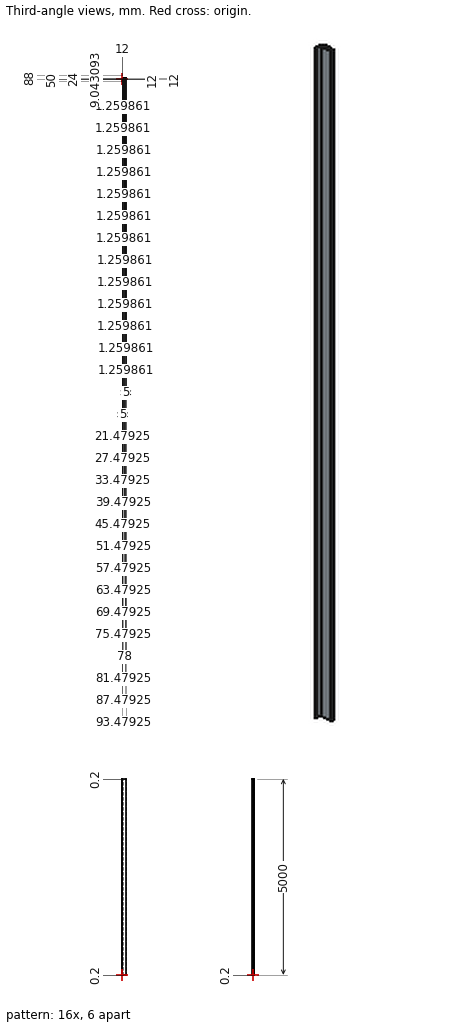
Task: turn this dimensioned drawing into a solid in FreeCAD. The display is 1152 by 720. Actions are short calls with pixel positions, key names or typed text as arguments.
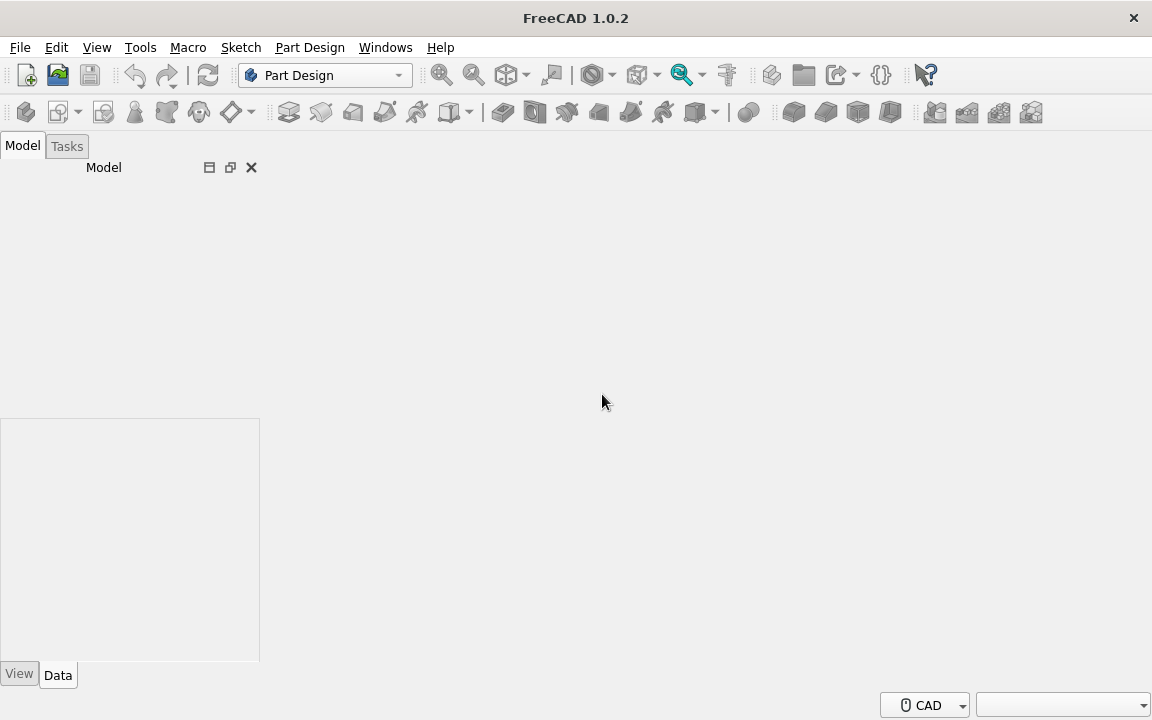
click(26, 76)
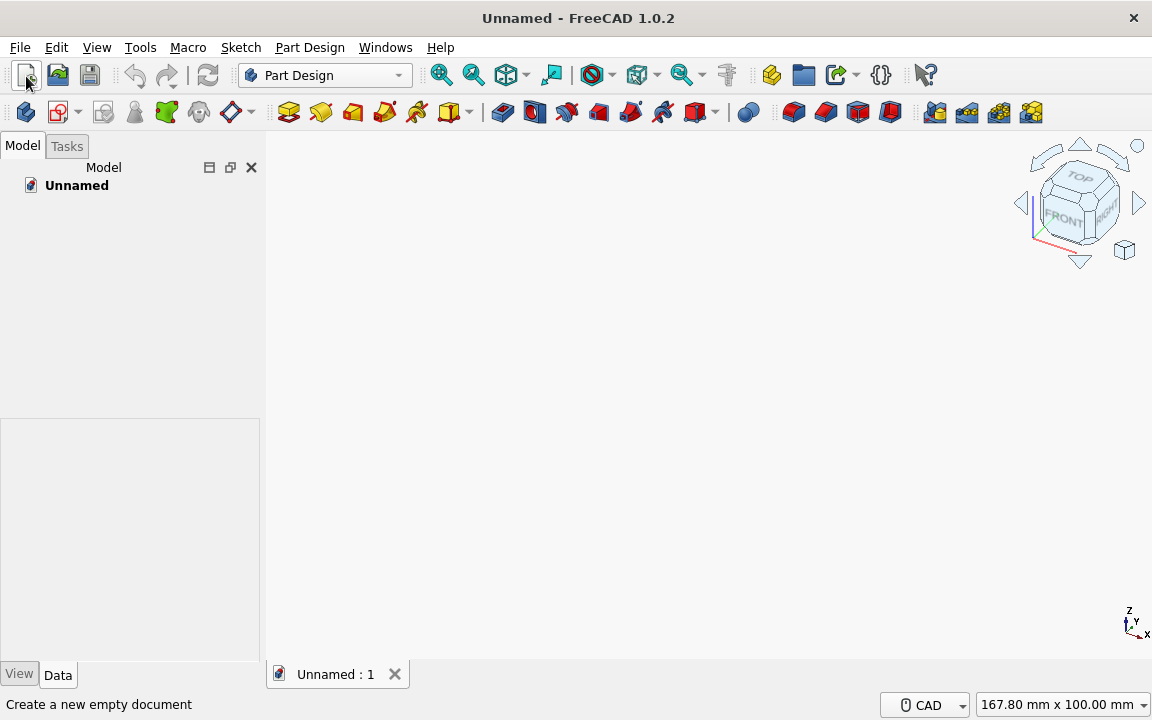
click(58, 112)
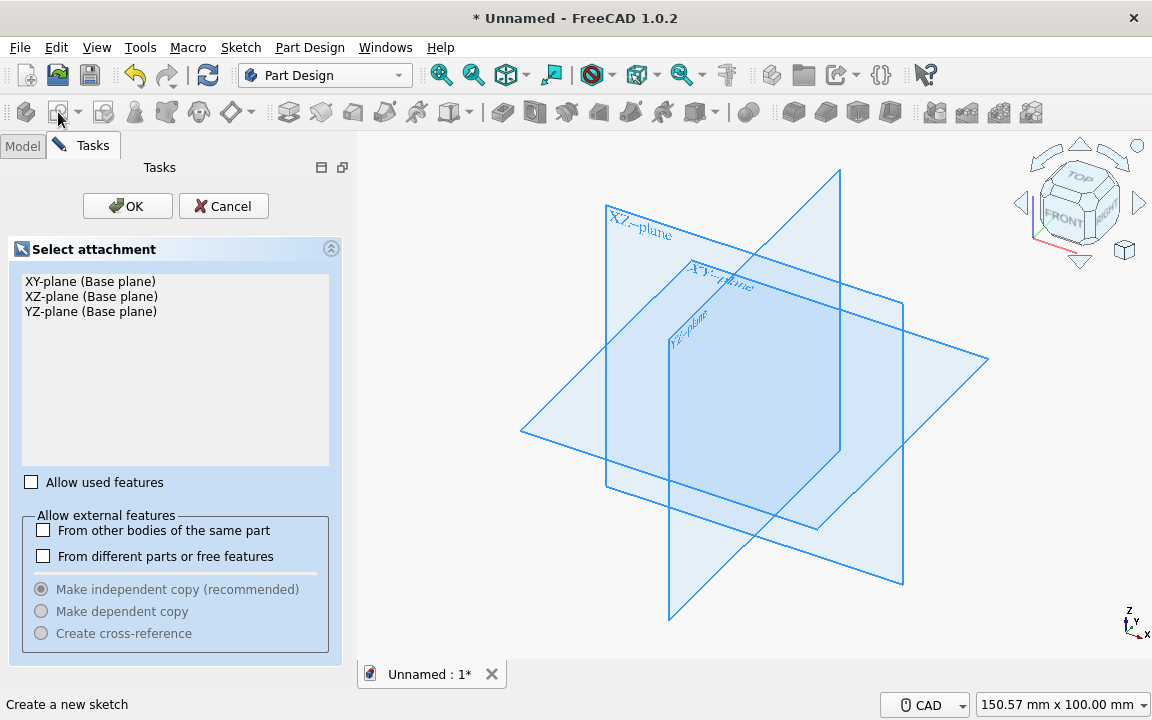
click(82, 282)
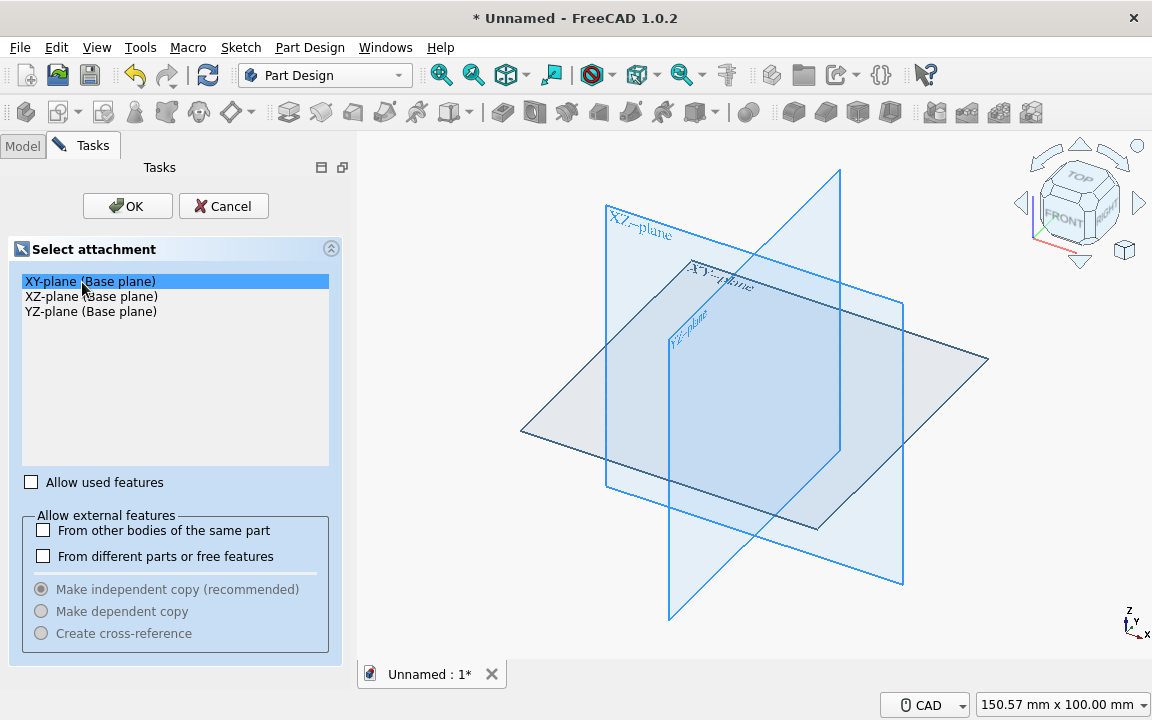
click(128, 206)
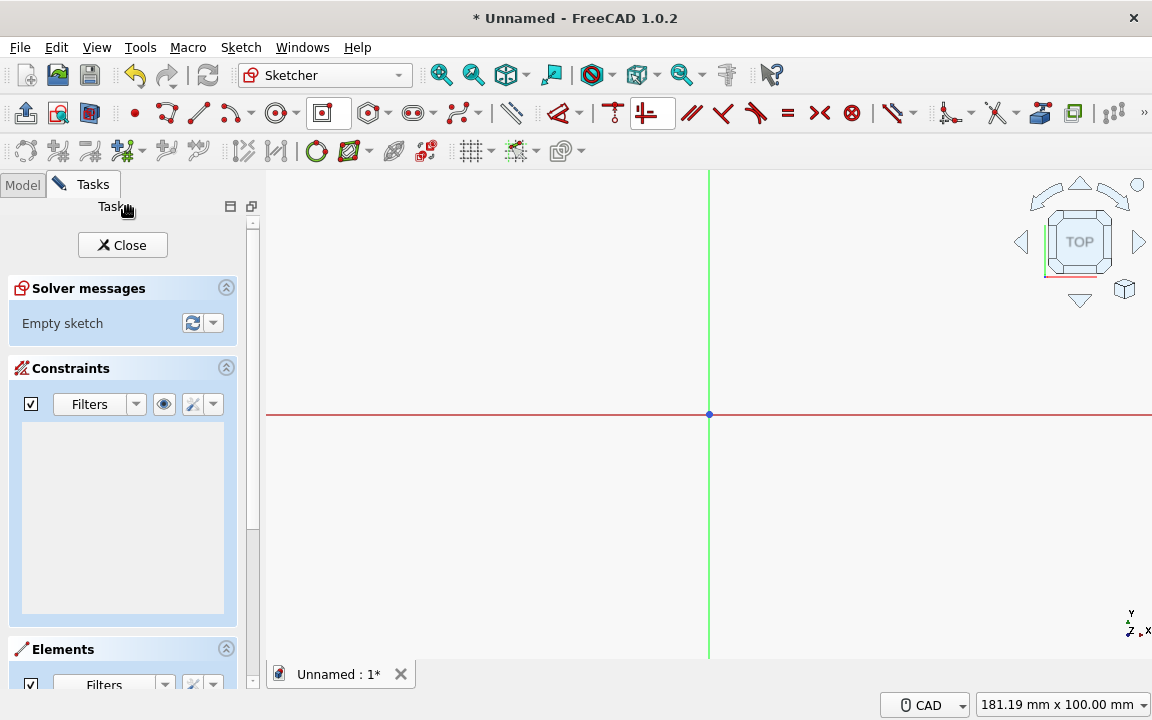
scroll(294, 631, down, 3)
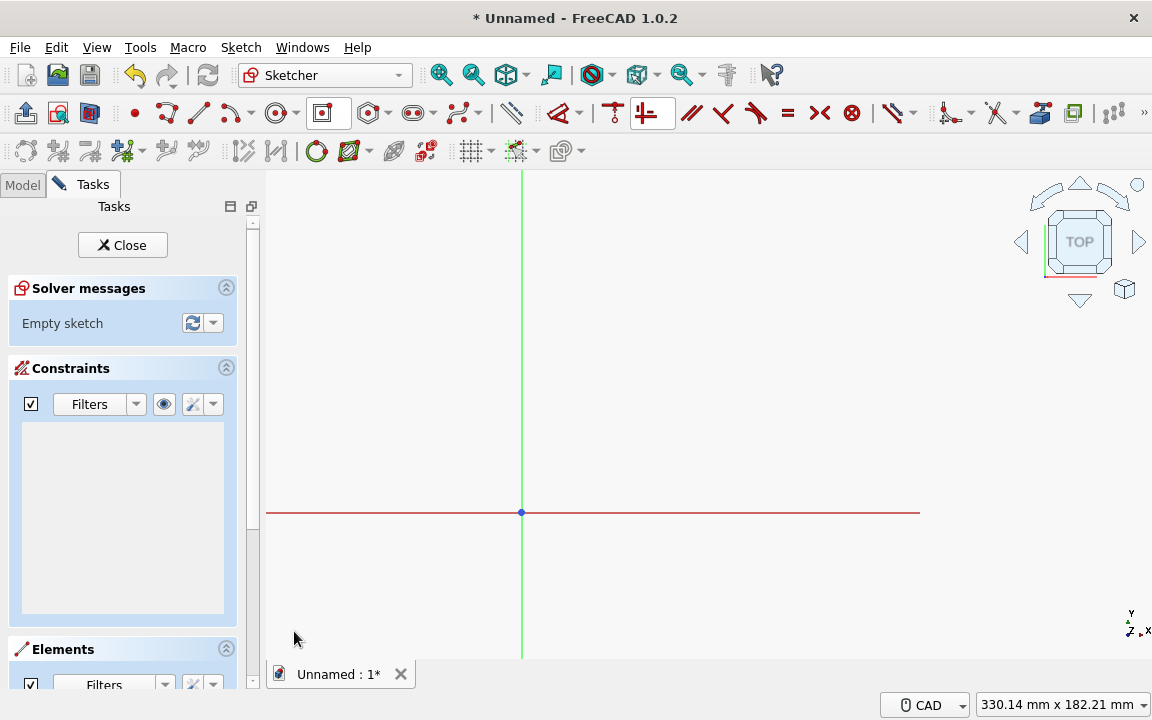
click(168, 114)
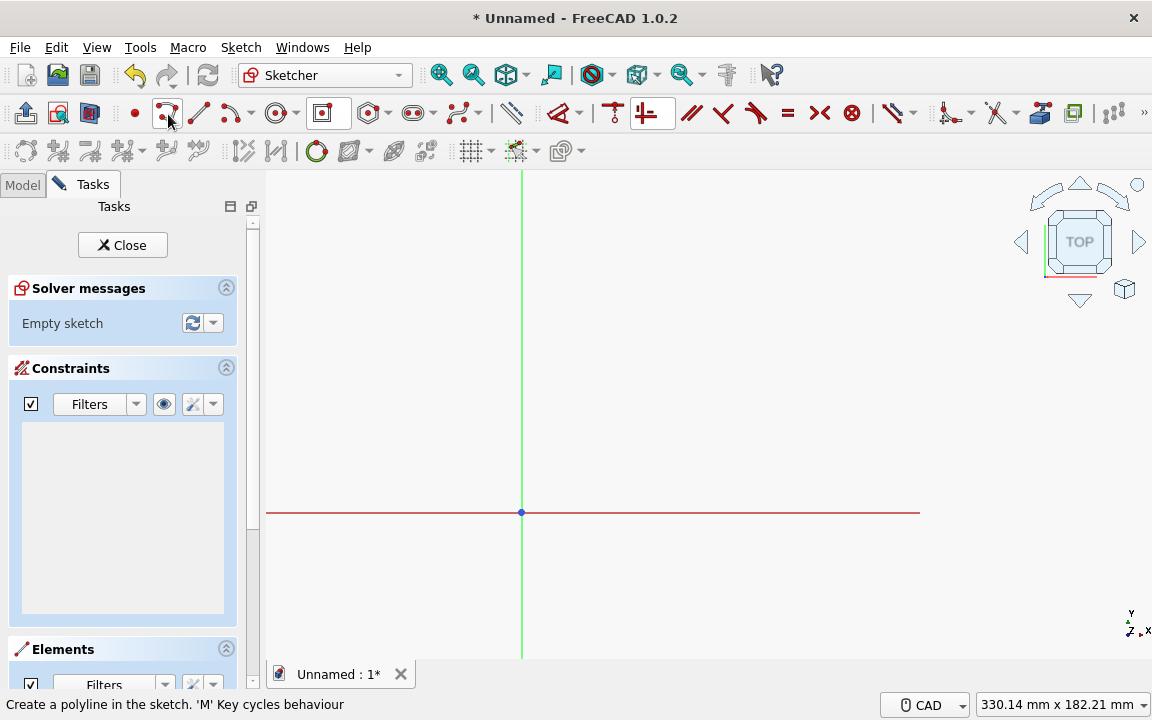
click(522, 513)
click(790, 504)
click(790, 480)
click(777, 480)
click(777, 448)
click(567, 448)
click(567, 480)
click(554, 480)
click(554, 244)
click(531, 244)
click(522, 513)
key(Escape)
key(Escape)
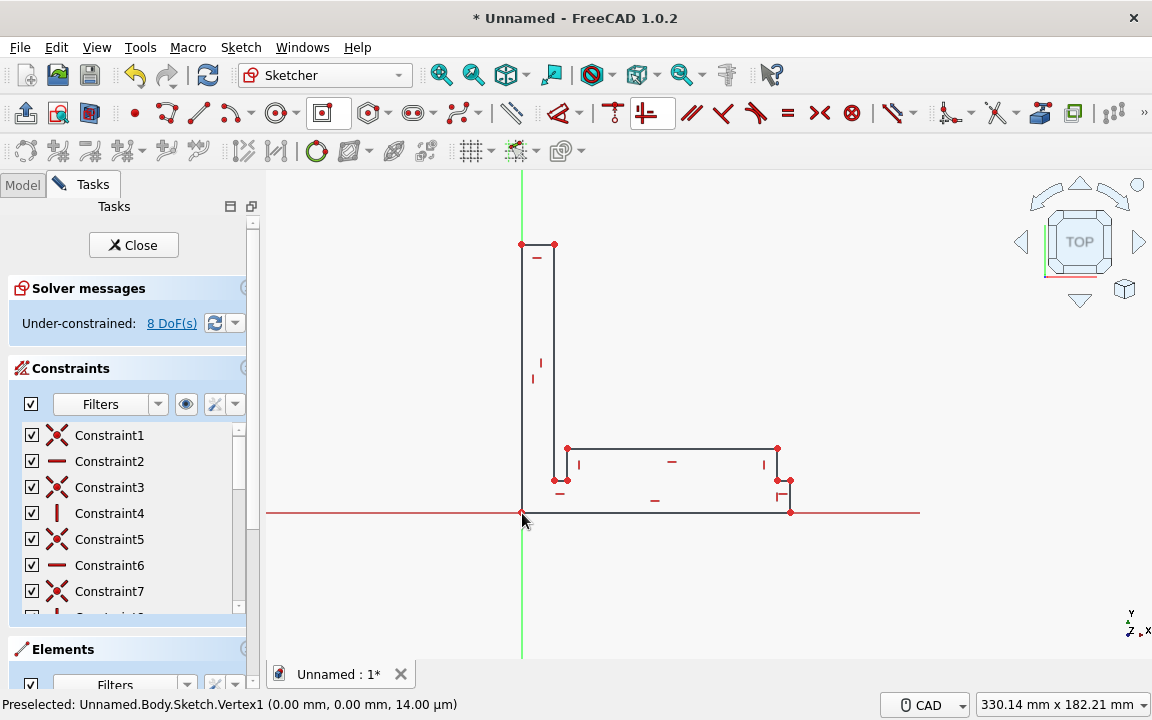
key(d)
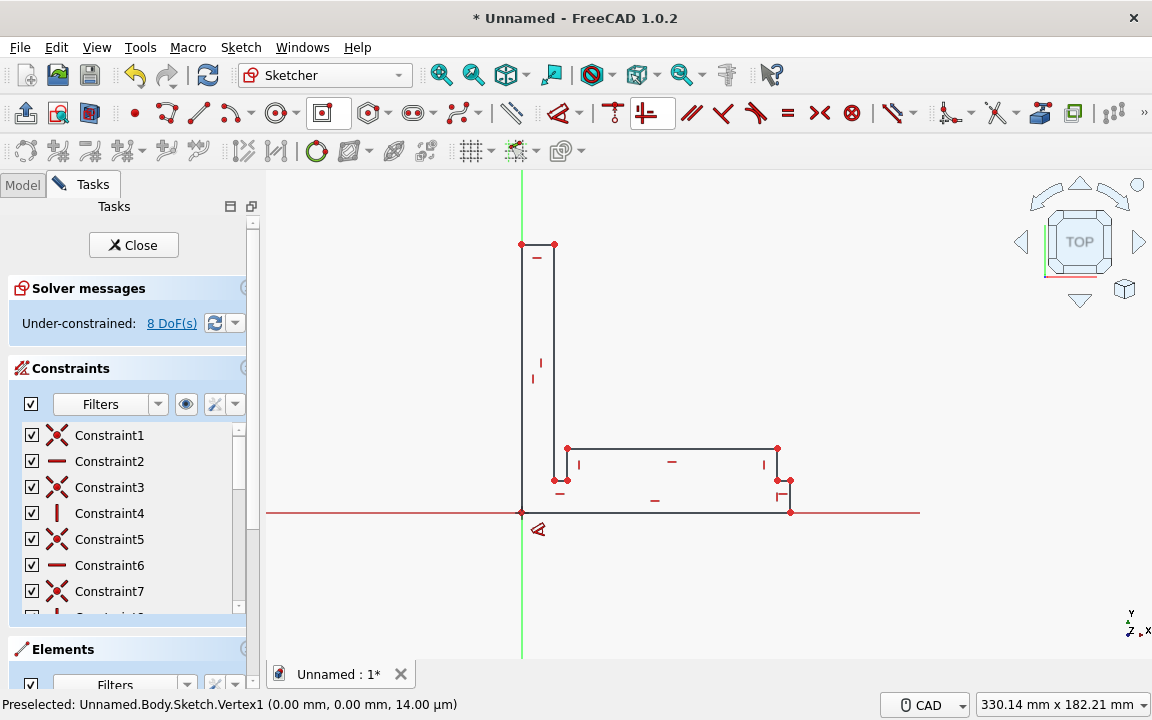
scroll(784, 481, up, 6)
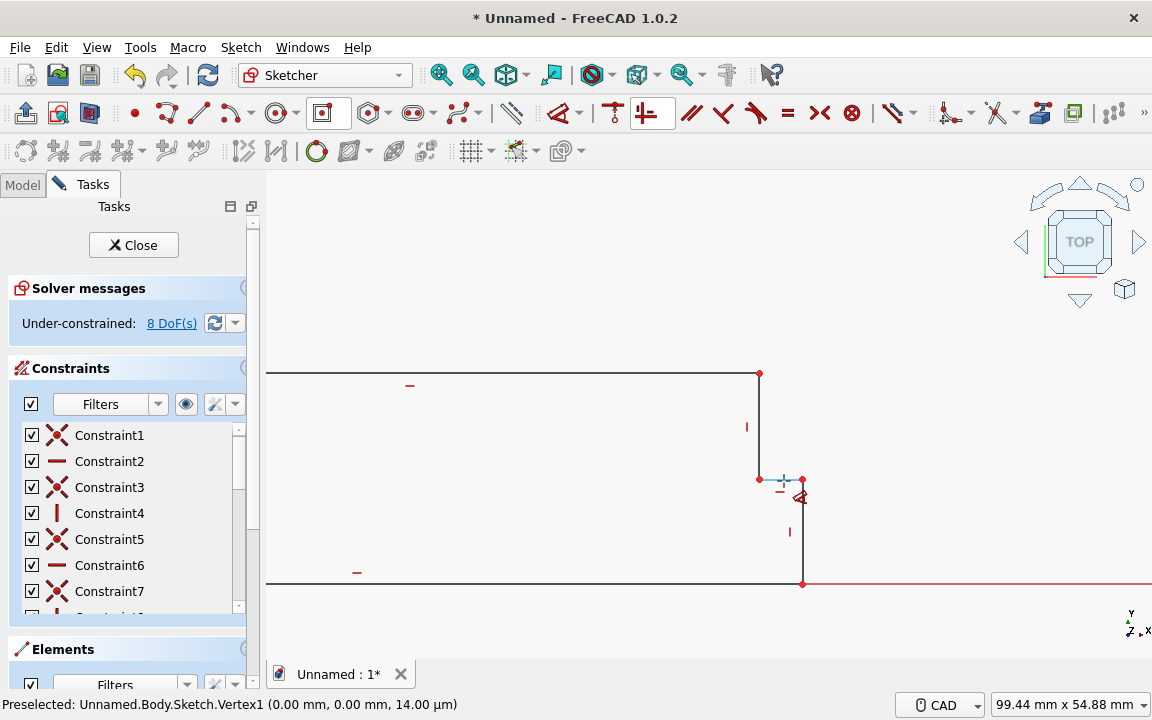
click(781, 480)
click(781, 514)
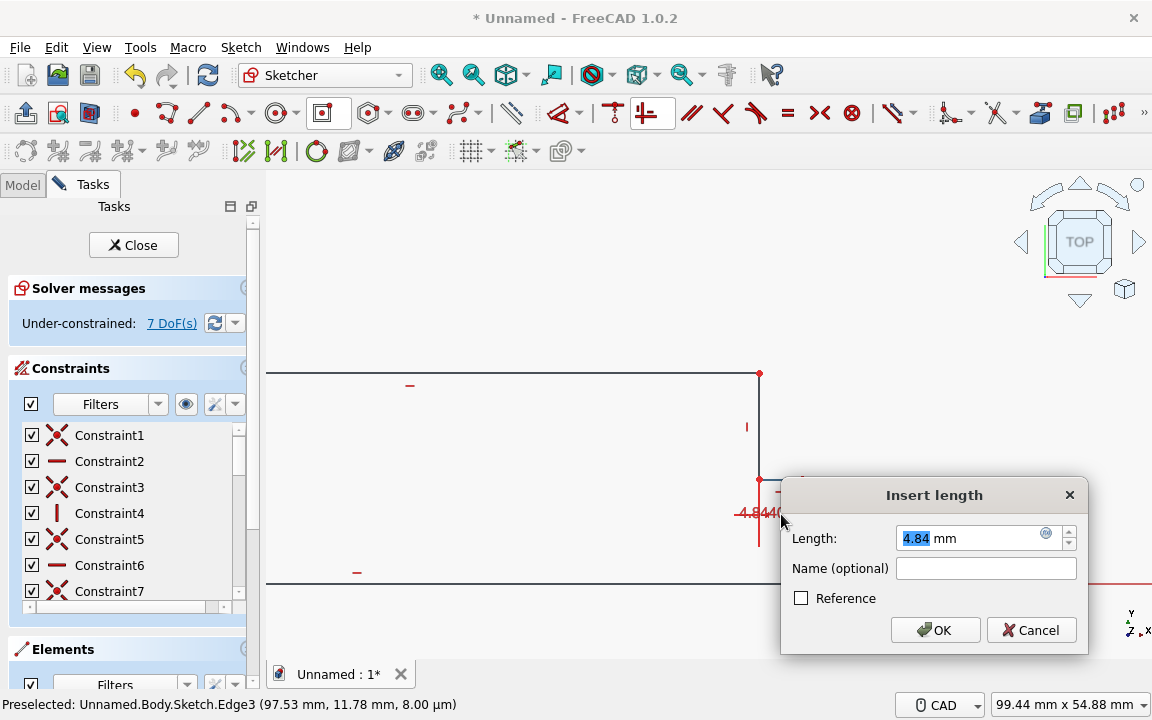
text(5)
key(Return)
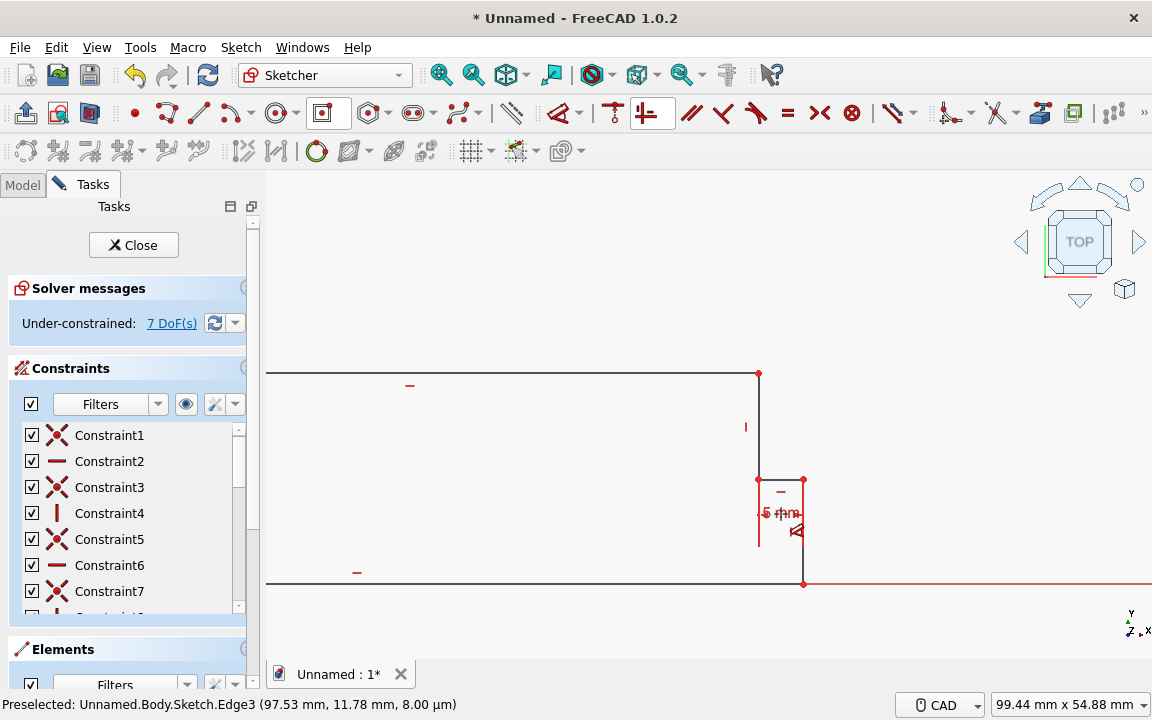
scroll(805, 575, down, 5)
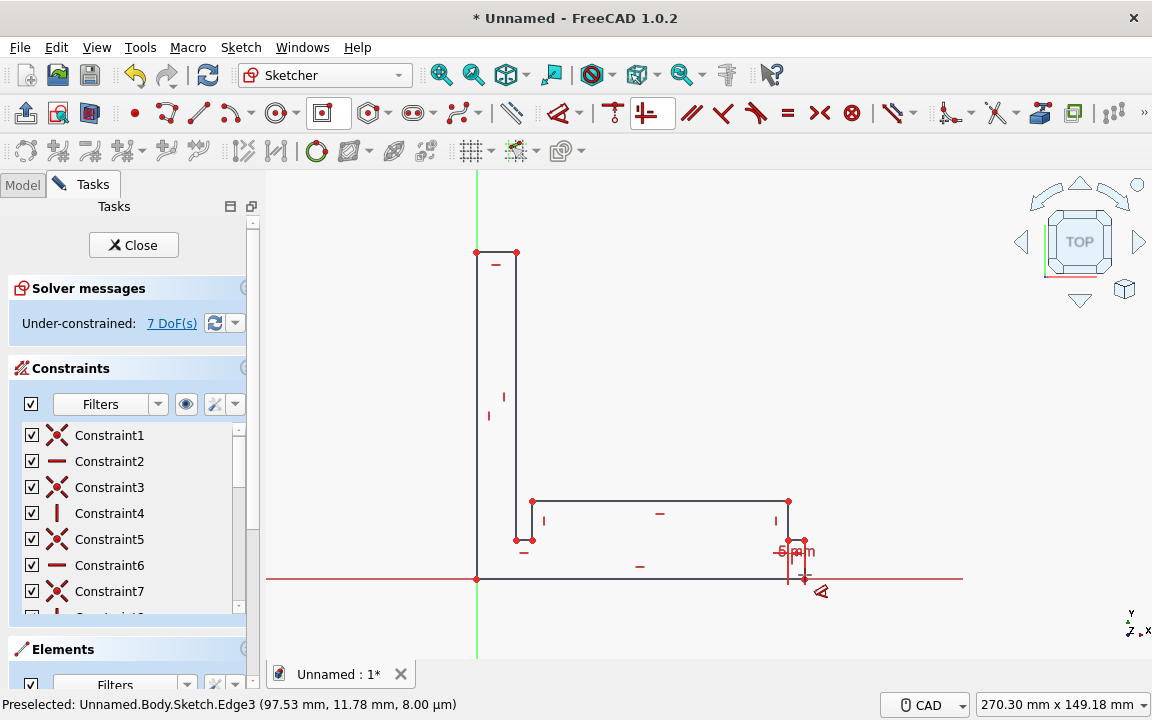
scroll(527, 540, up, 6)